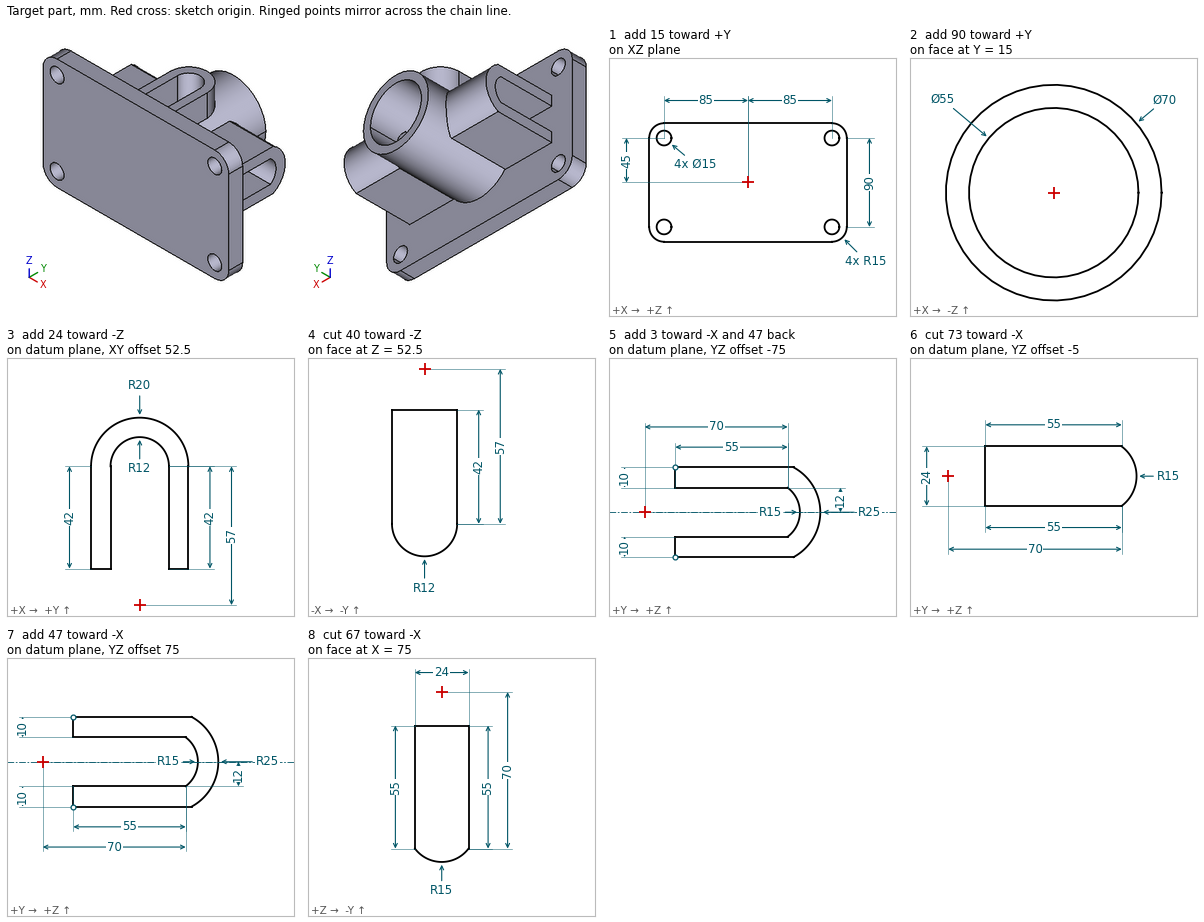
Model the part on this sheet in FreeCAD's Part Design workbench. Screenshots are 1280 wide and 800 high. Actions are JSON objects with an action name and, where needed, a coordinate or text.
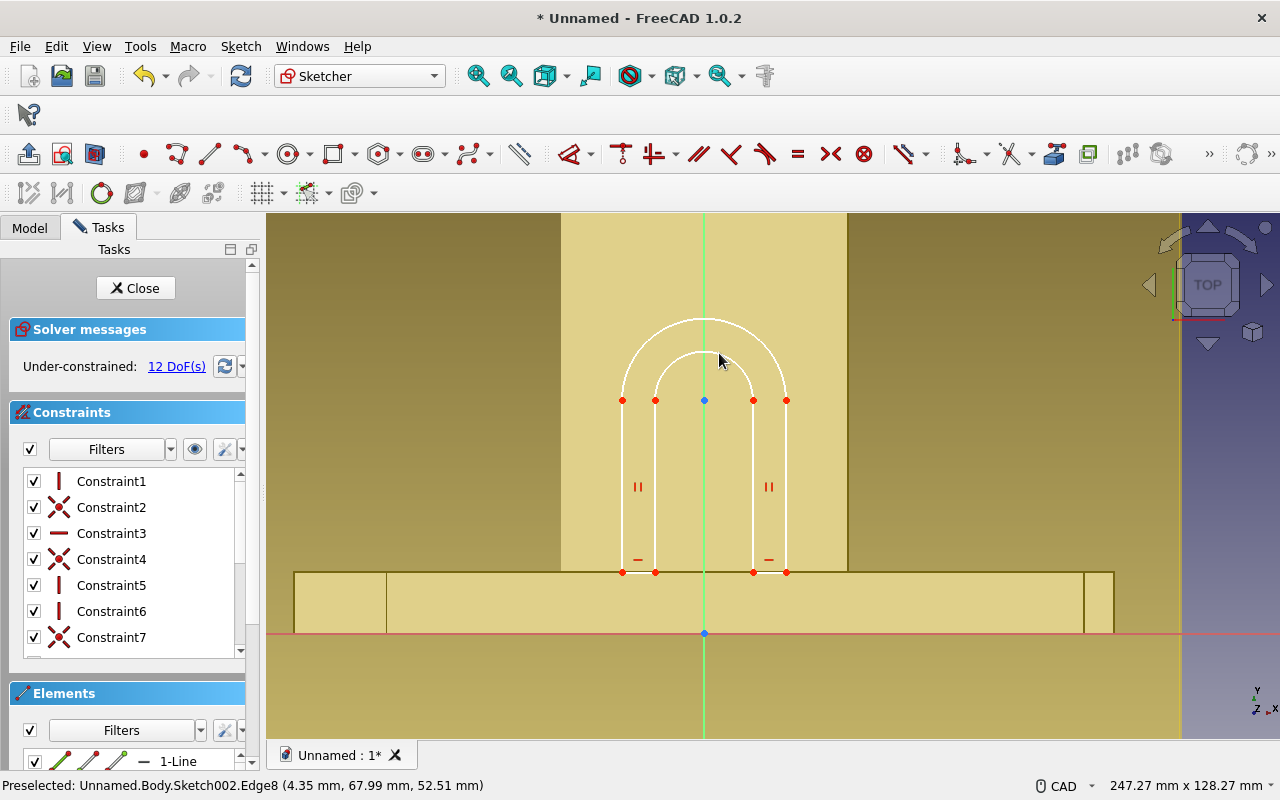
{"action": "left_click", "coordinate": [753, 453]}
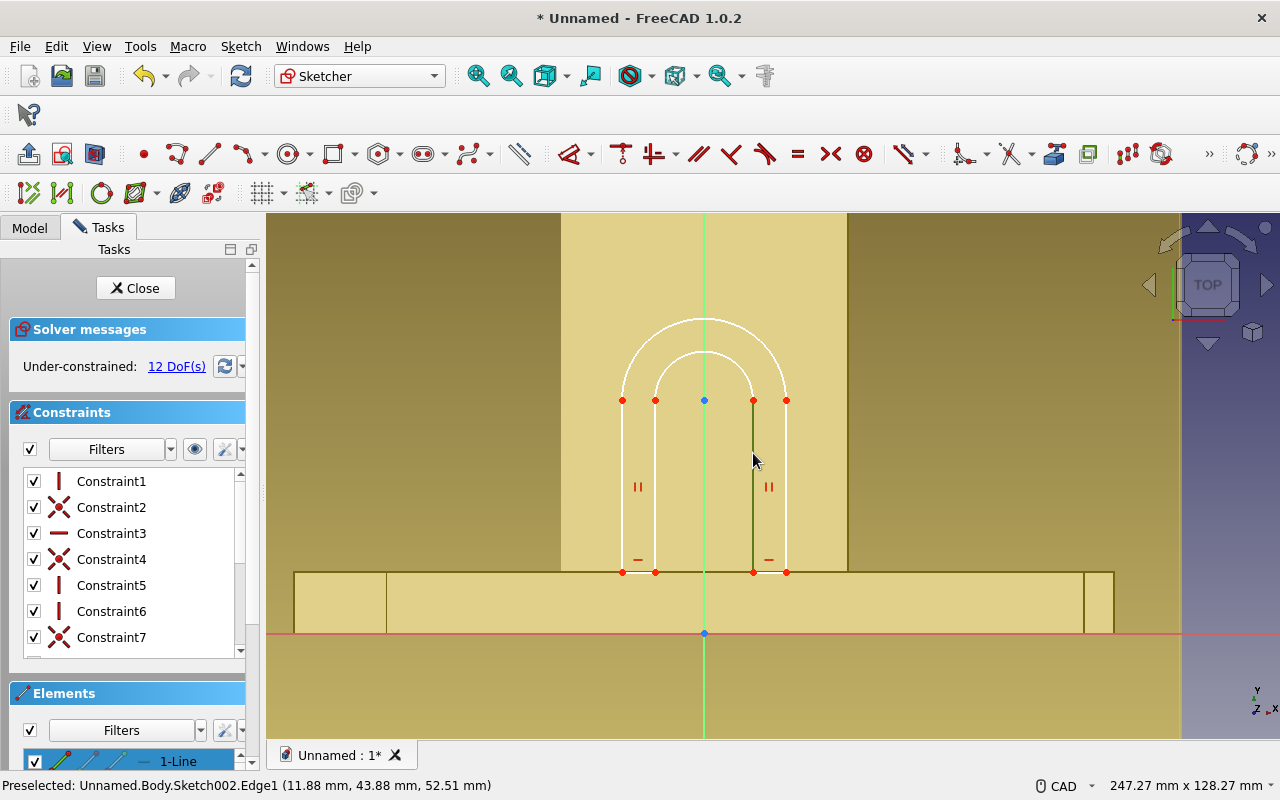
{"action": "left_click", "coordinate": [733, 361]}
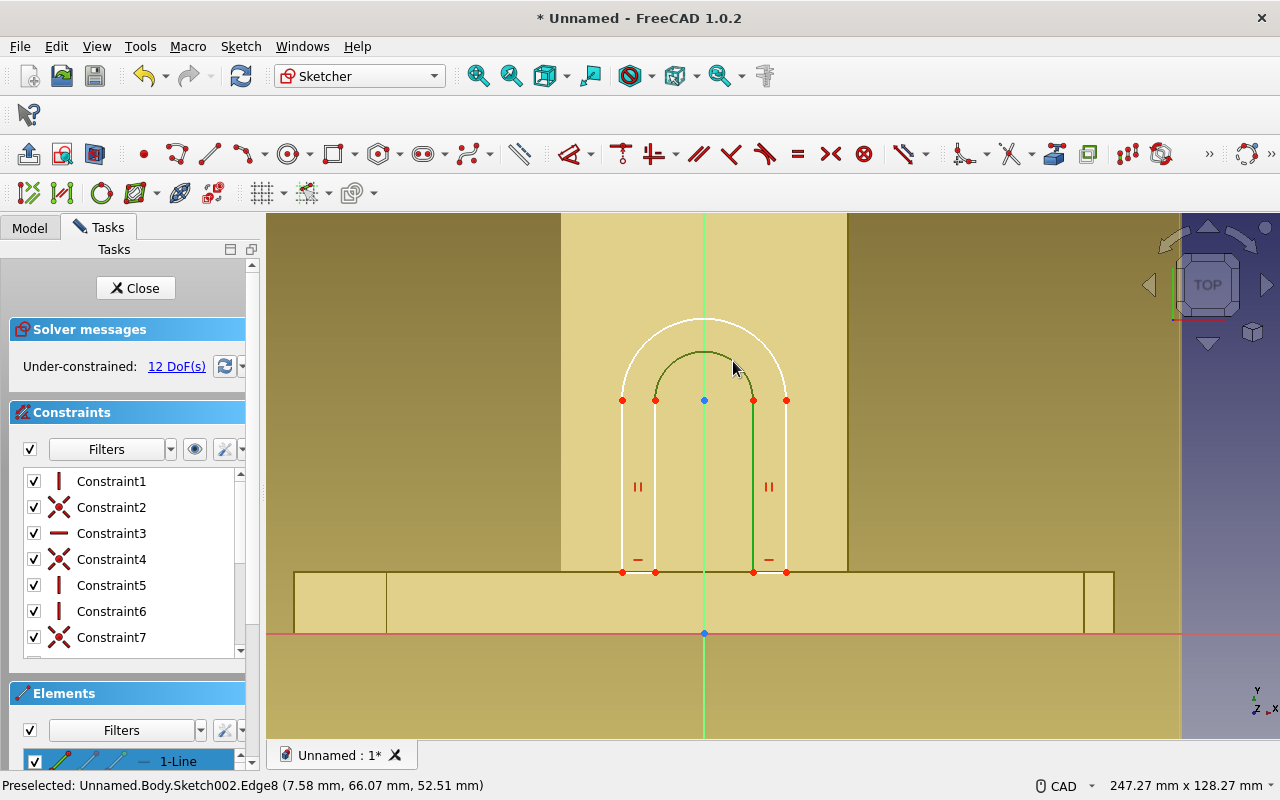
{"action": "key", "text": "t"}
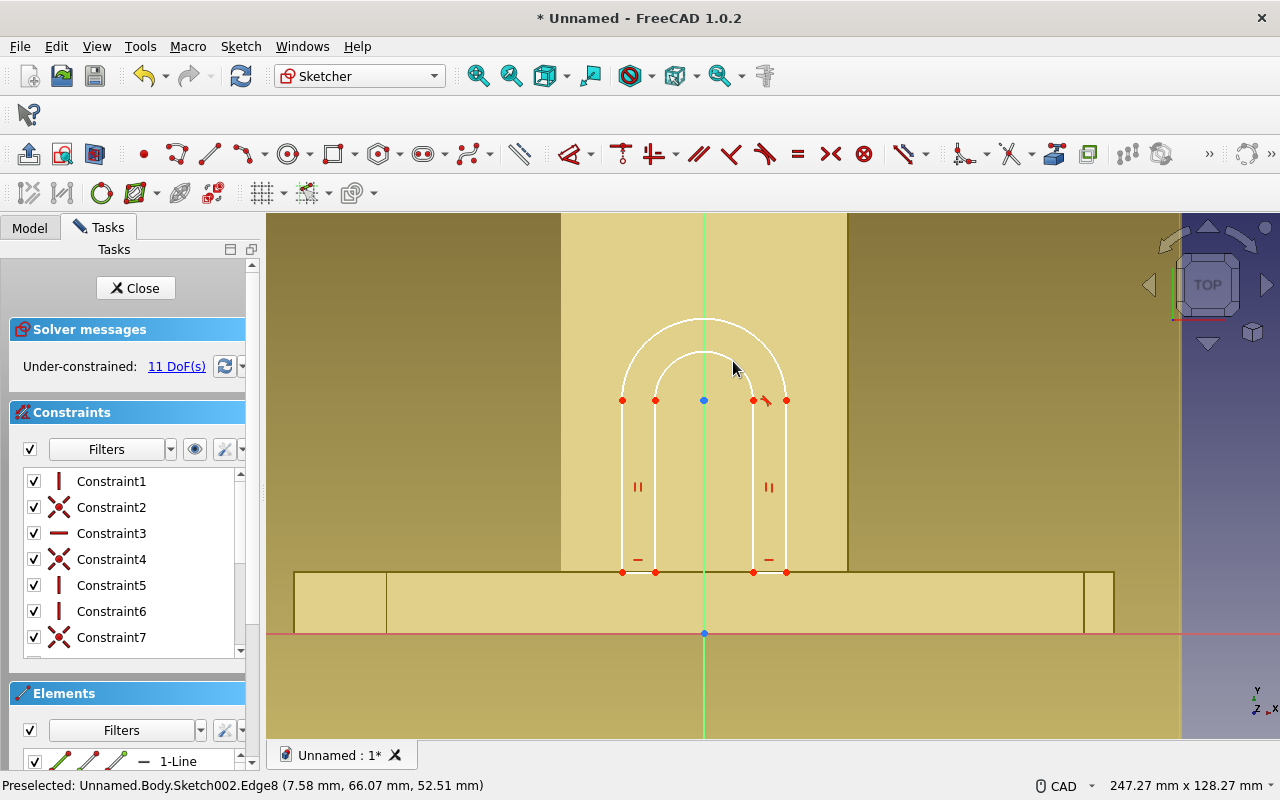
{"action": "left_click", "coordinate": [786, 521]}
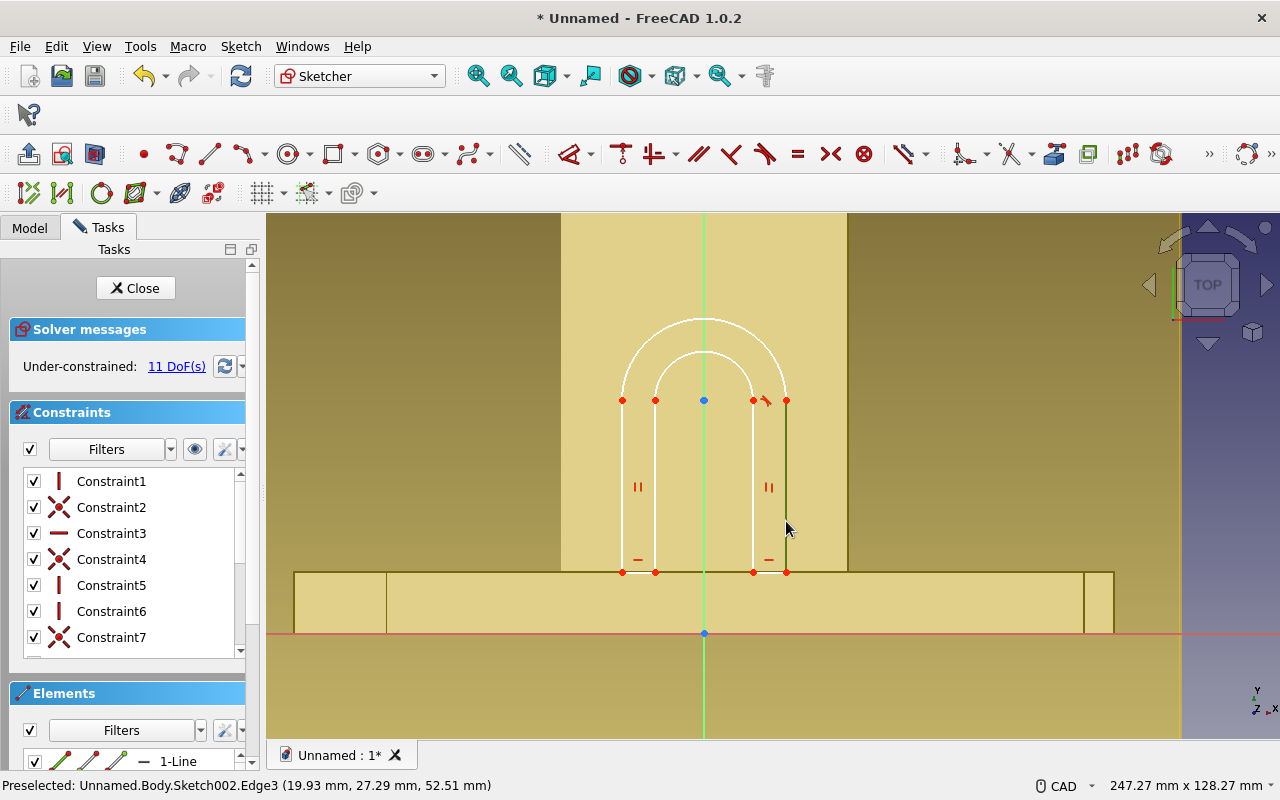
{"action": "left_click", "coordinate": [752, 334]}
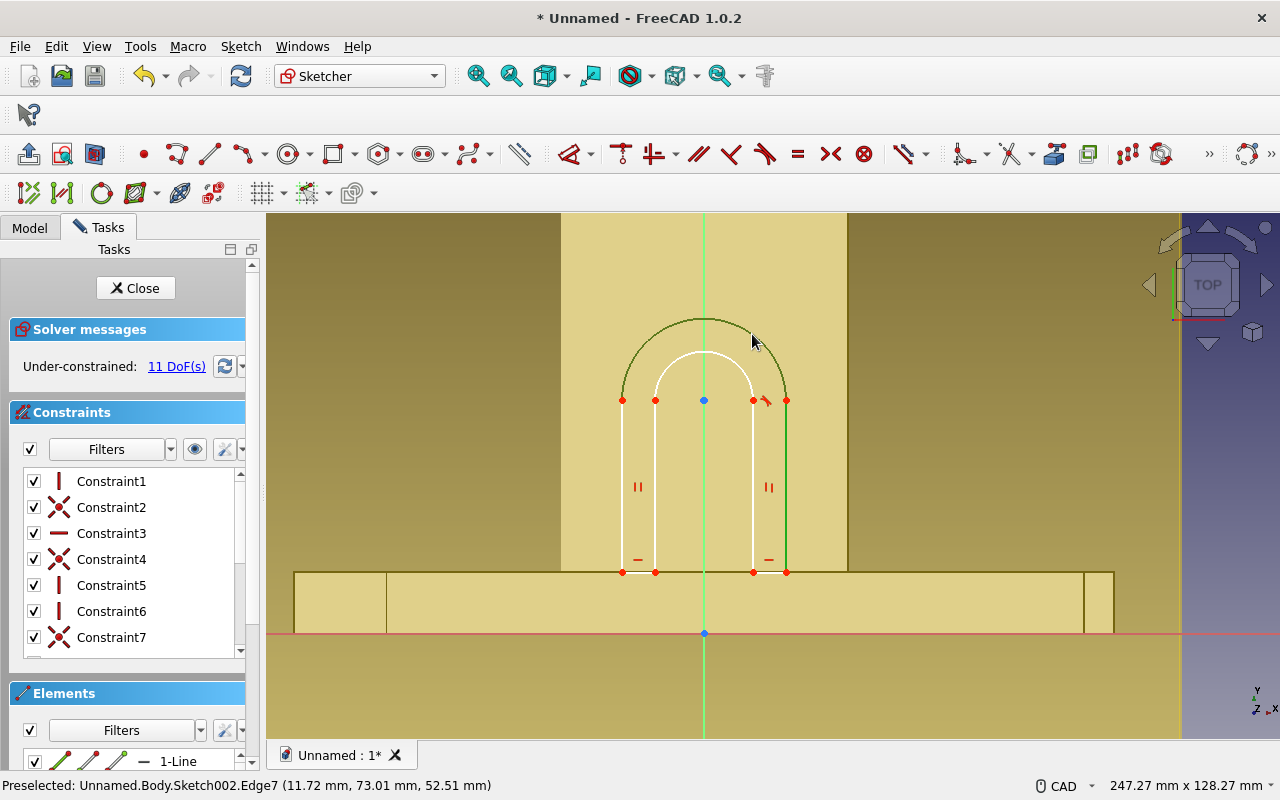
{"action": "left_click", "coordinate": [765, 154]}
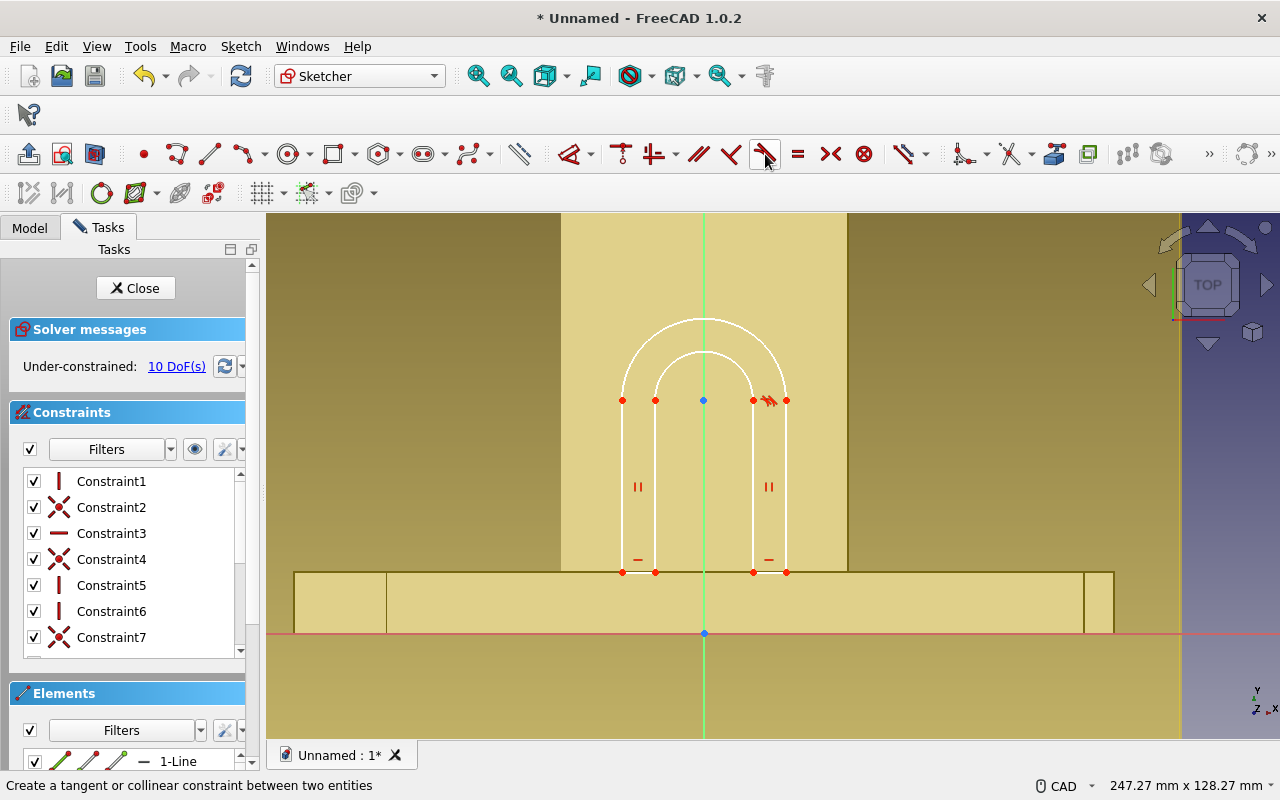
{"action": "left_click", "coordinate": [622, 453]}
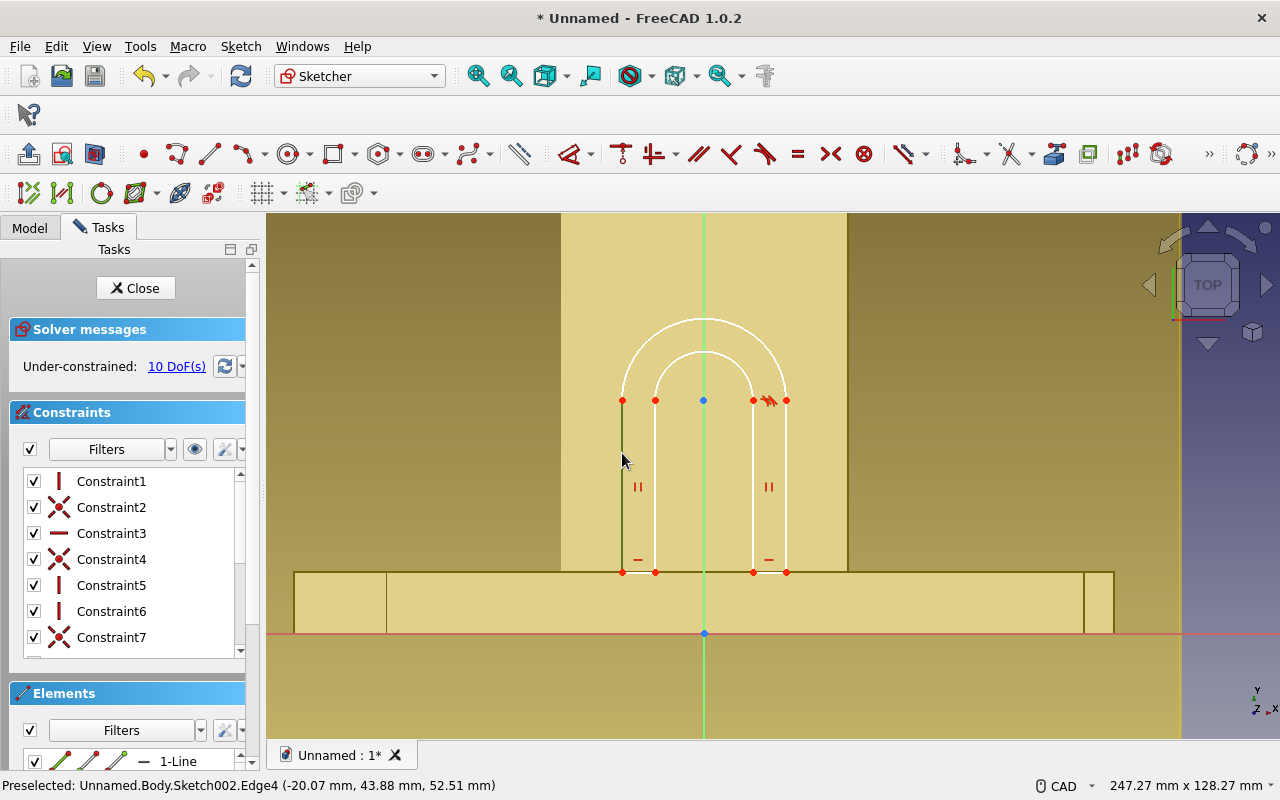
{"action": "left_click", "coordinate": [752, 334]}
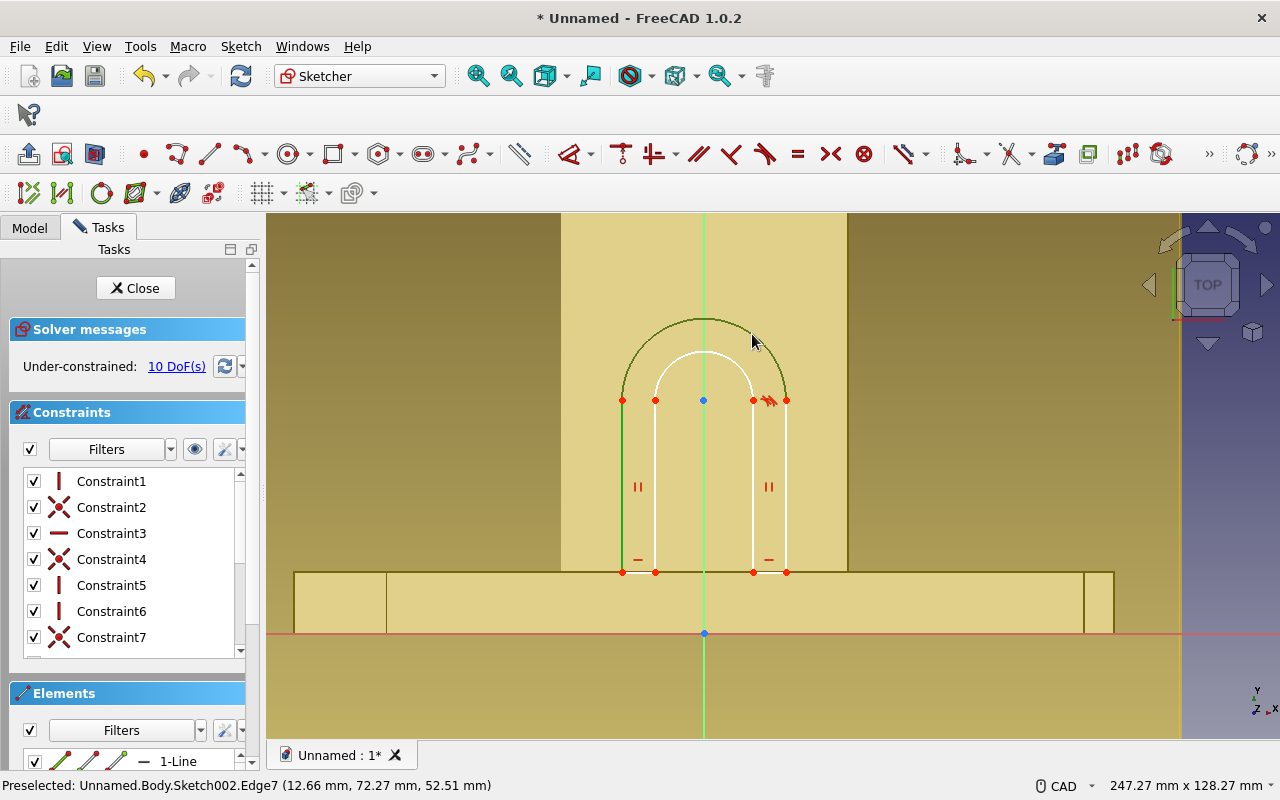
{"action": "left_click", "coordinate": [765, 154]}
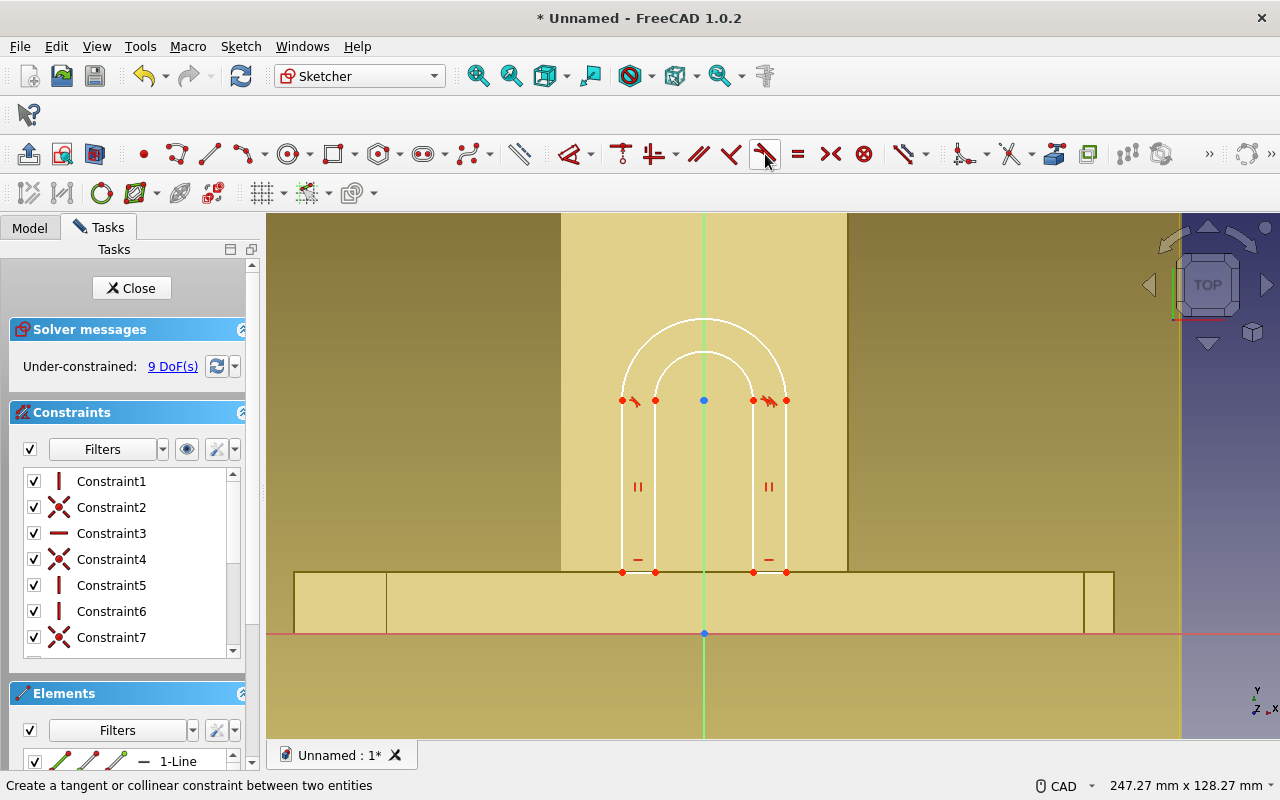
{"action": "left_click", "coordinate": [655, 521]}